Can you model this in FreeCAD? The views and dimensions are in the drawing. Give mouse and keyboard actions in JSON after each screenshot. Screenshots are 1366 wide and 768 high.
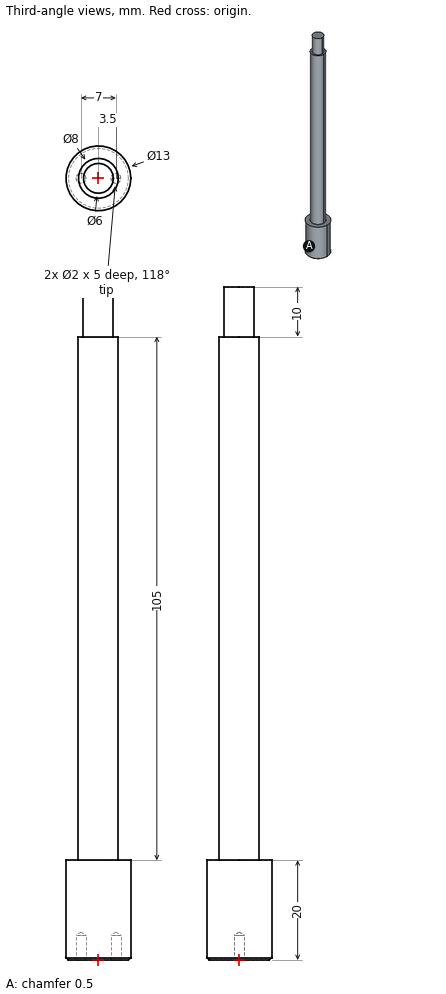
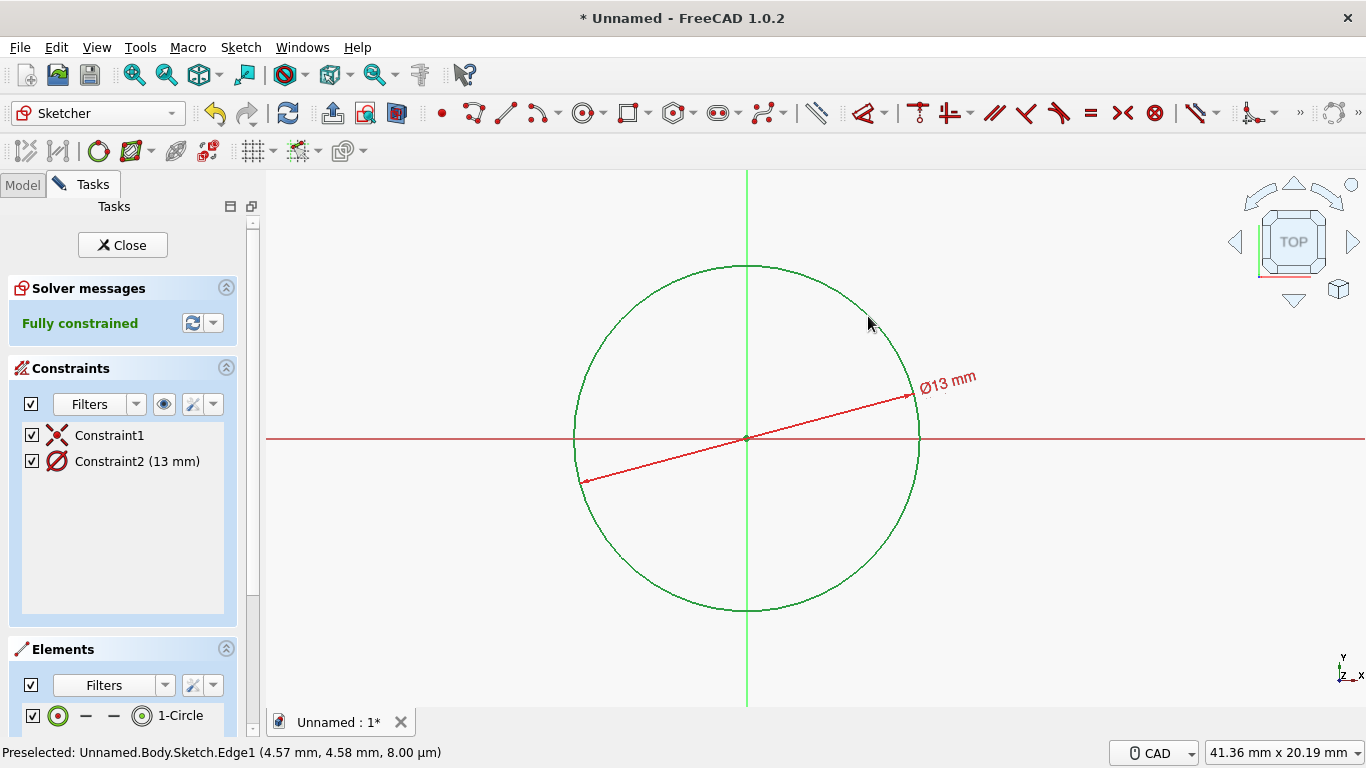
{"action": "left_click", "coordinate": [123, 245]}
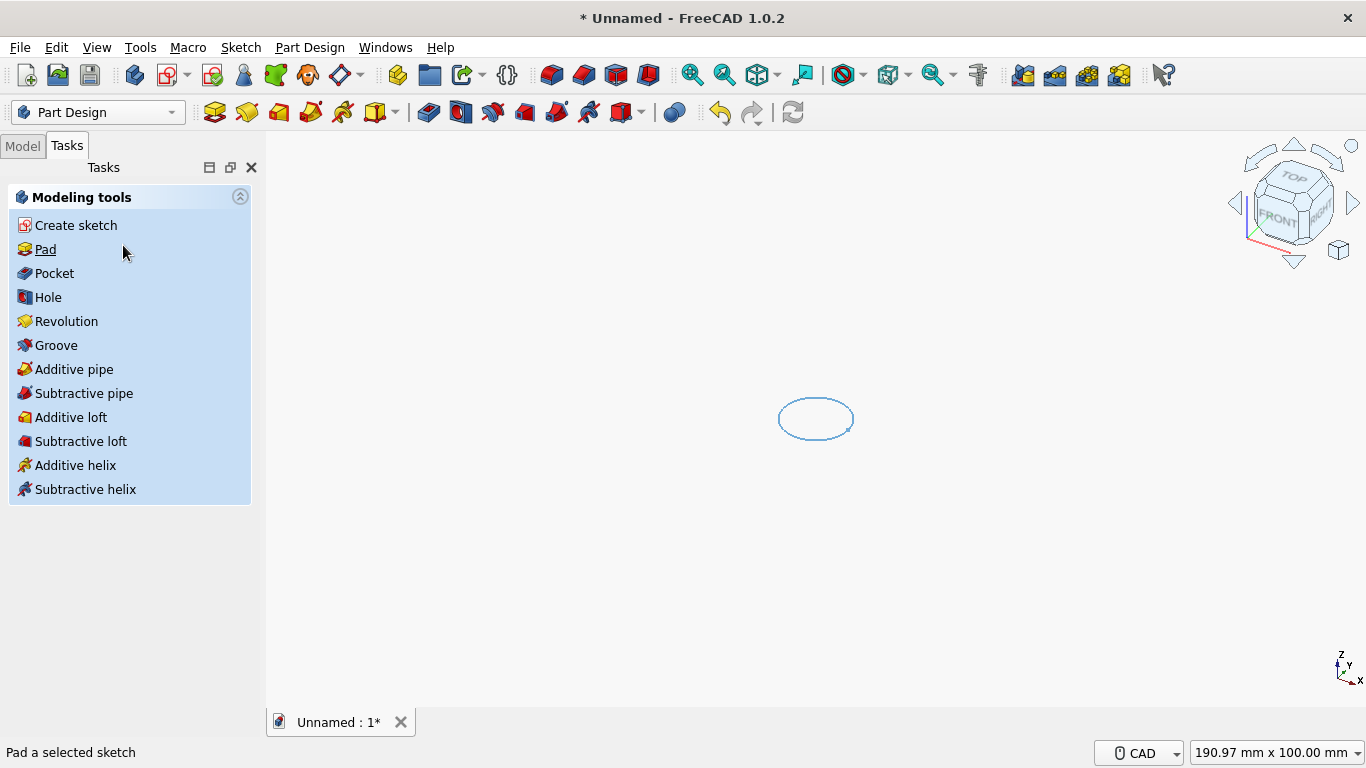
{"action": "left_click", "coordinate": [216, 112]}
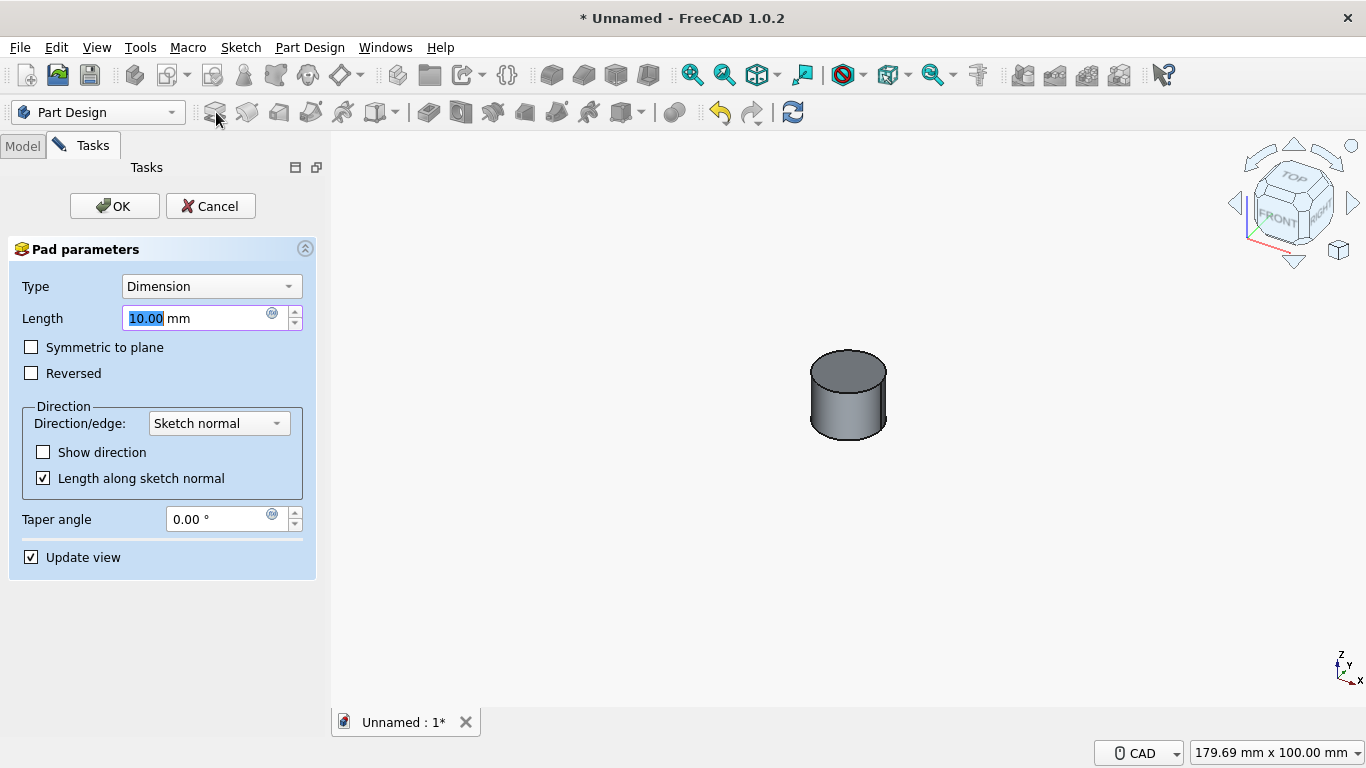
{"action": "type", "text": "20"}
{"action": "key", "text": "Tab"}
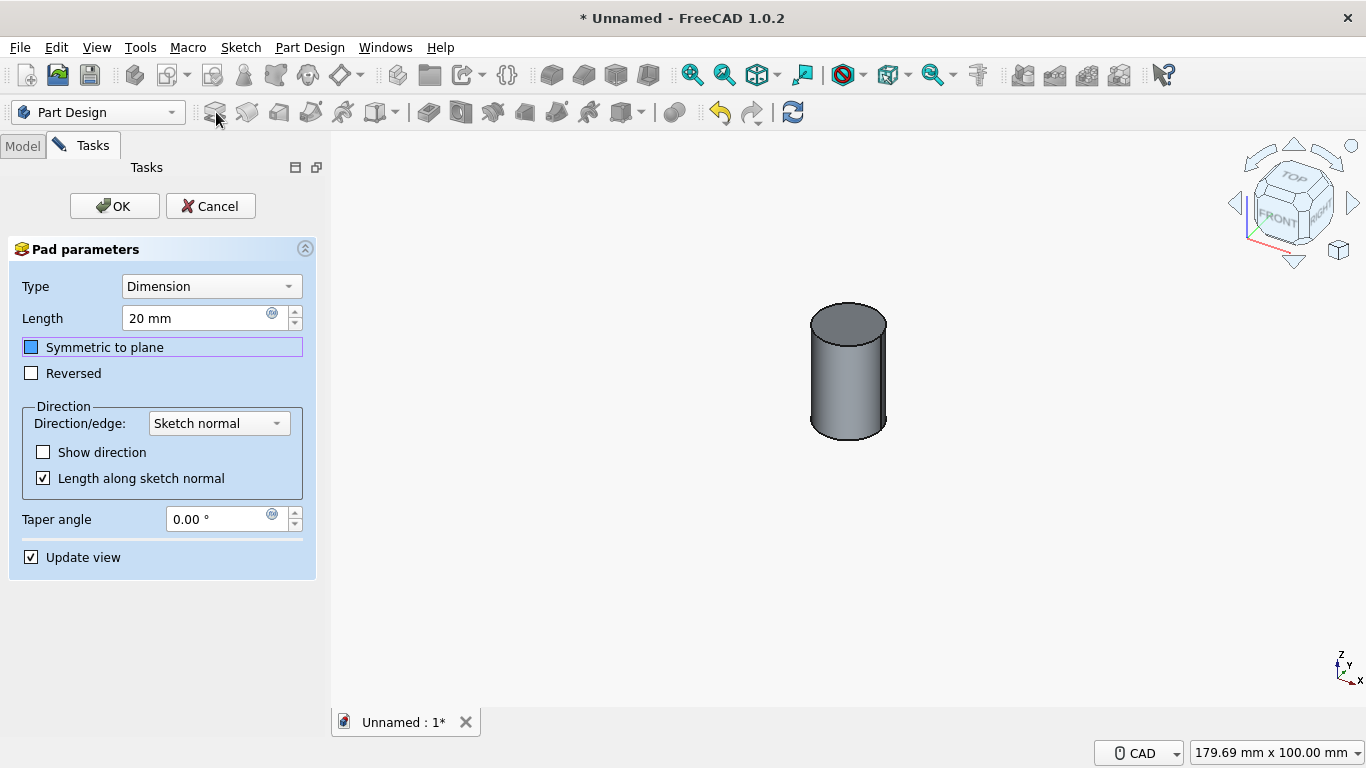
{"action": "left_click", "coordinate": [115, 206]}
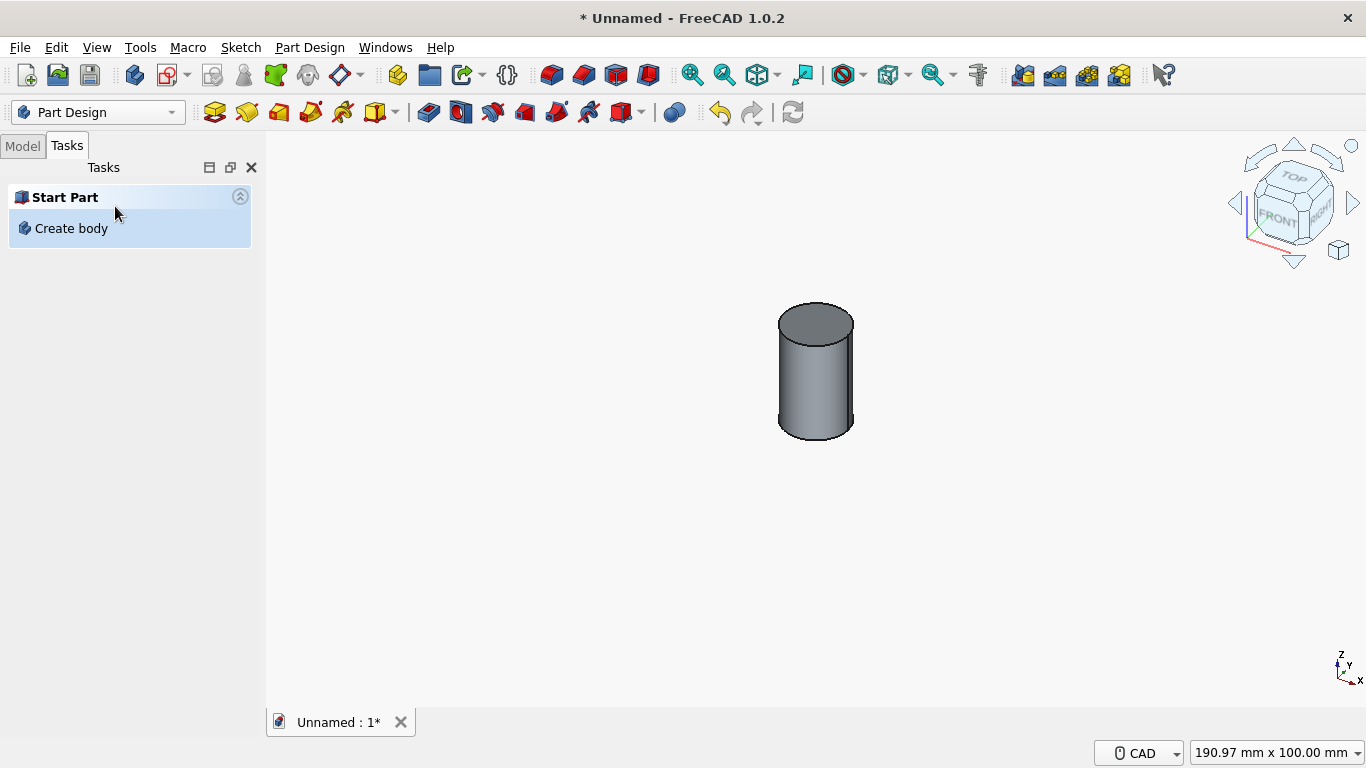
{"action": "left_click", "coordinate": [694, 76]}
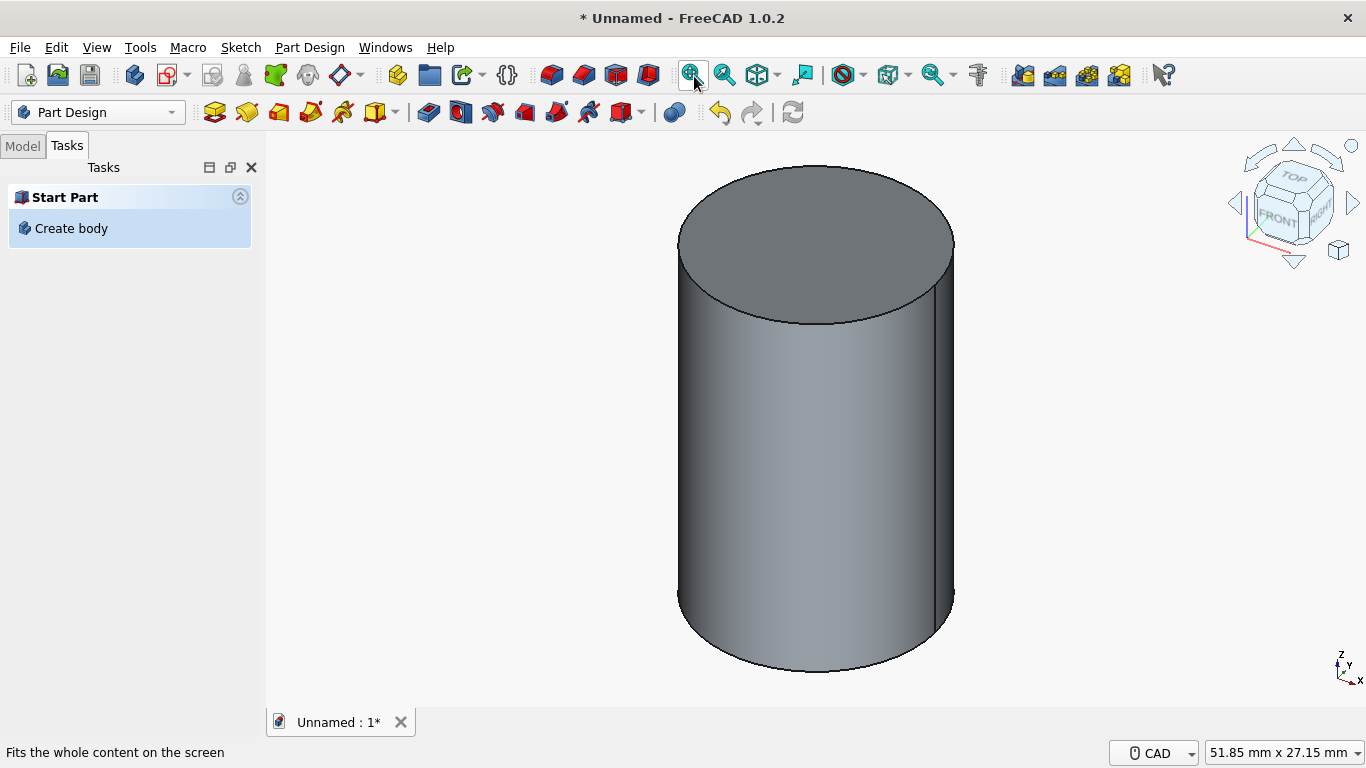
{"action": "key", "text": "0"}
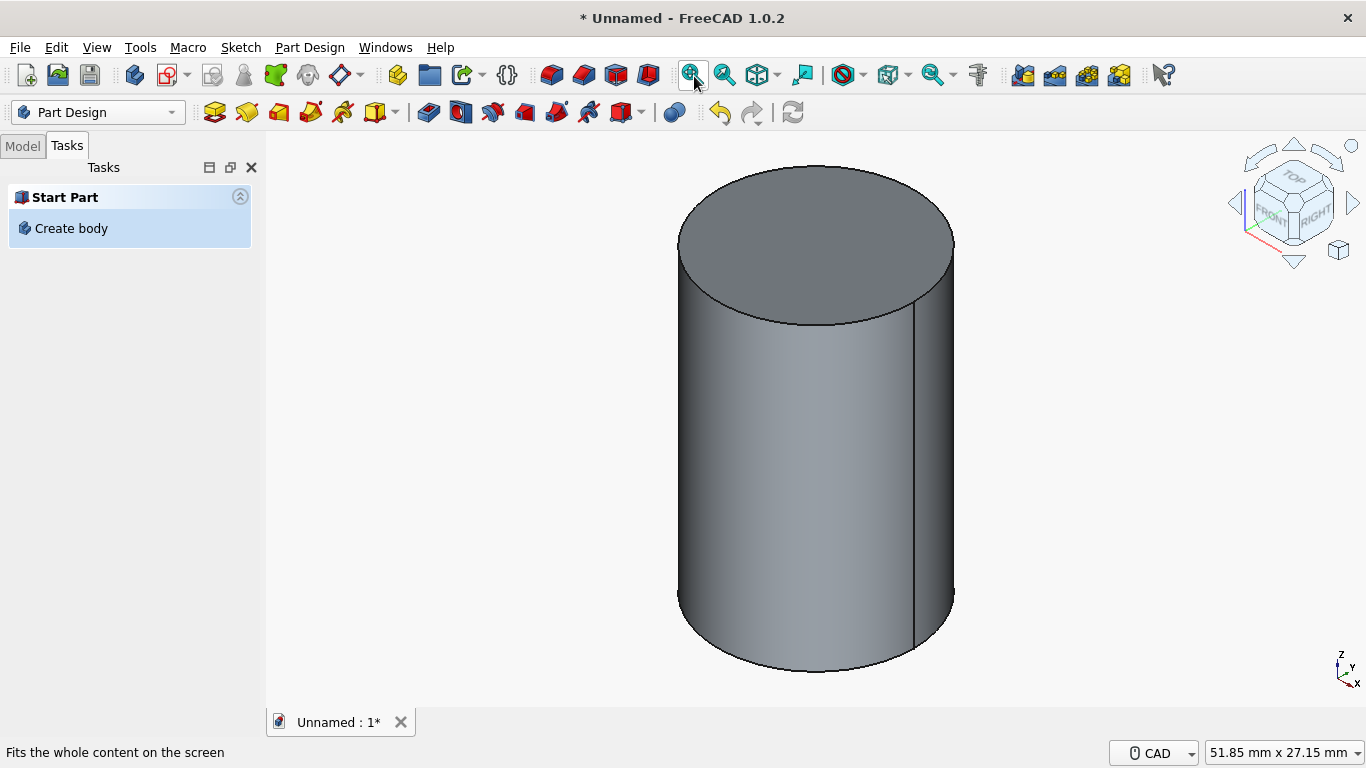
{"action": "key", "text": "2"}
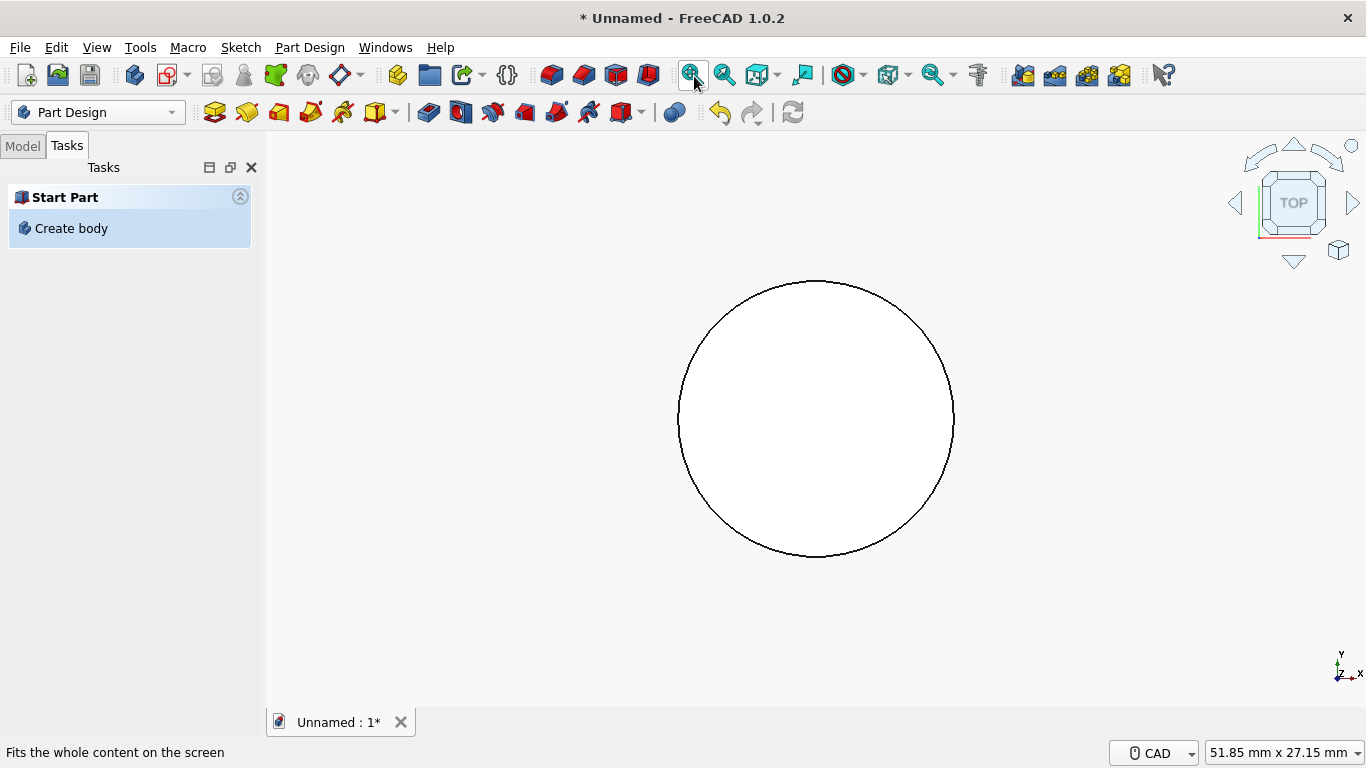
{"action": "key", "text": "1"}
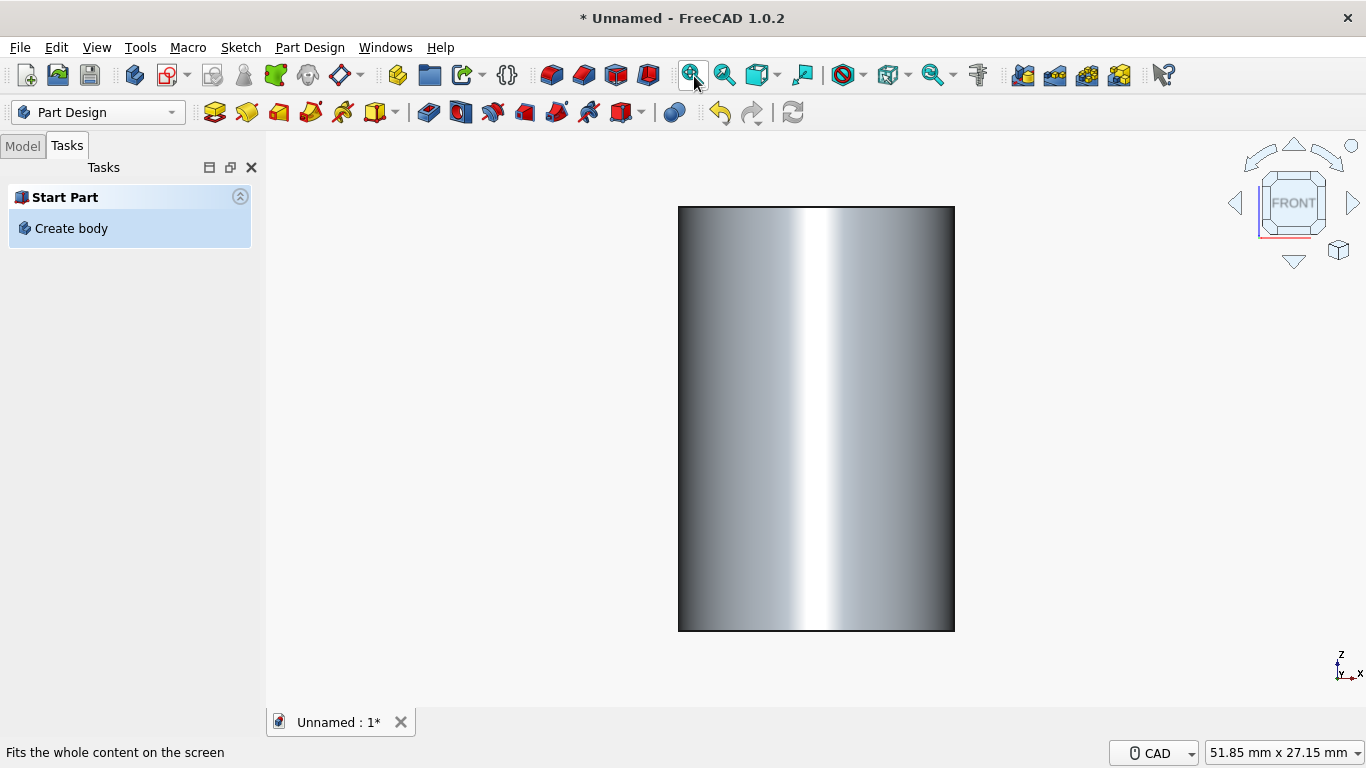
{"action": "left_click", "coordinate": [704, 630]}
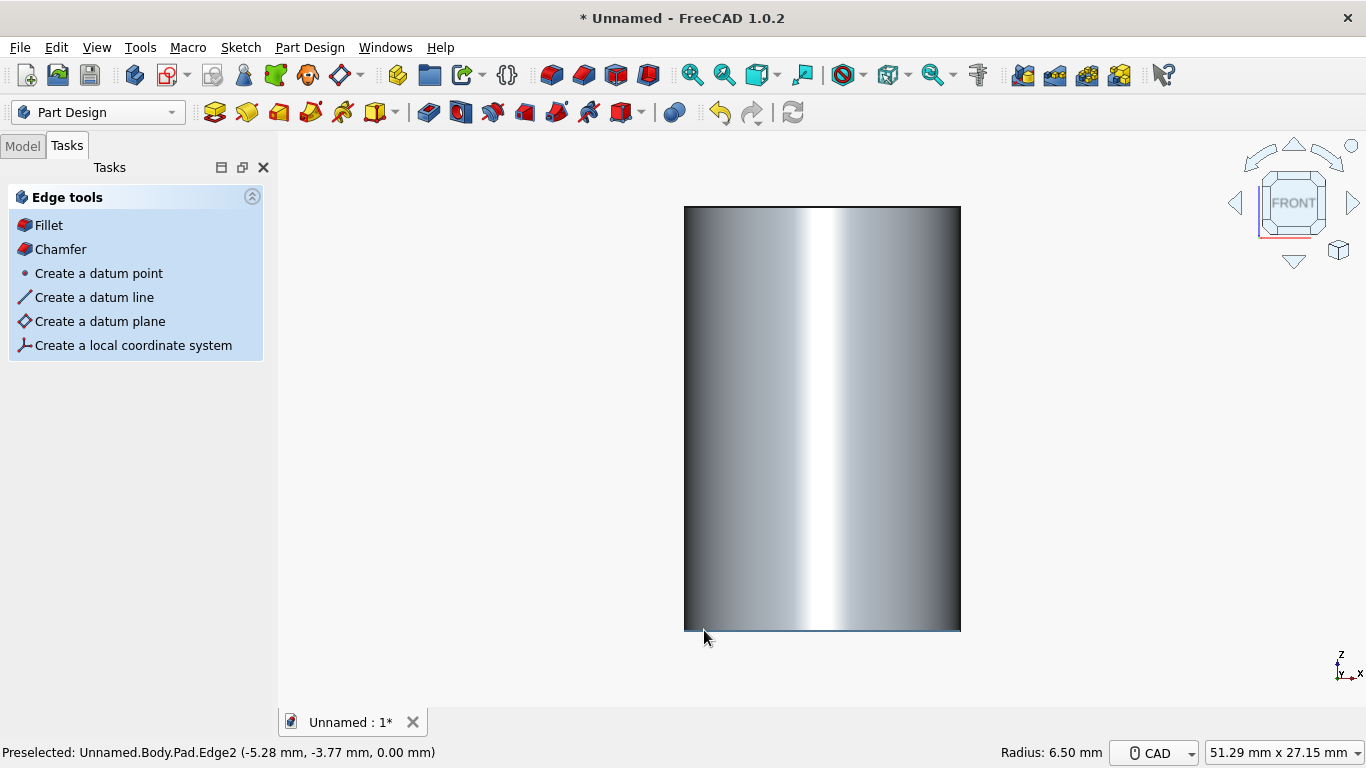
{"action": "left_click", "coordinate": [584, 76]}